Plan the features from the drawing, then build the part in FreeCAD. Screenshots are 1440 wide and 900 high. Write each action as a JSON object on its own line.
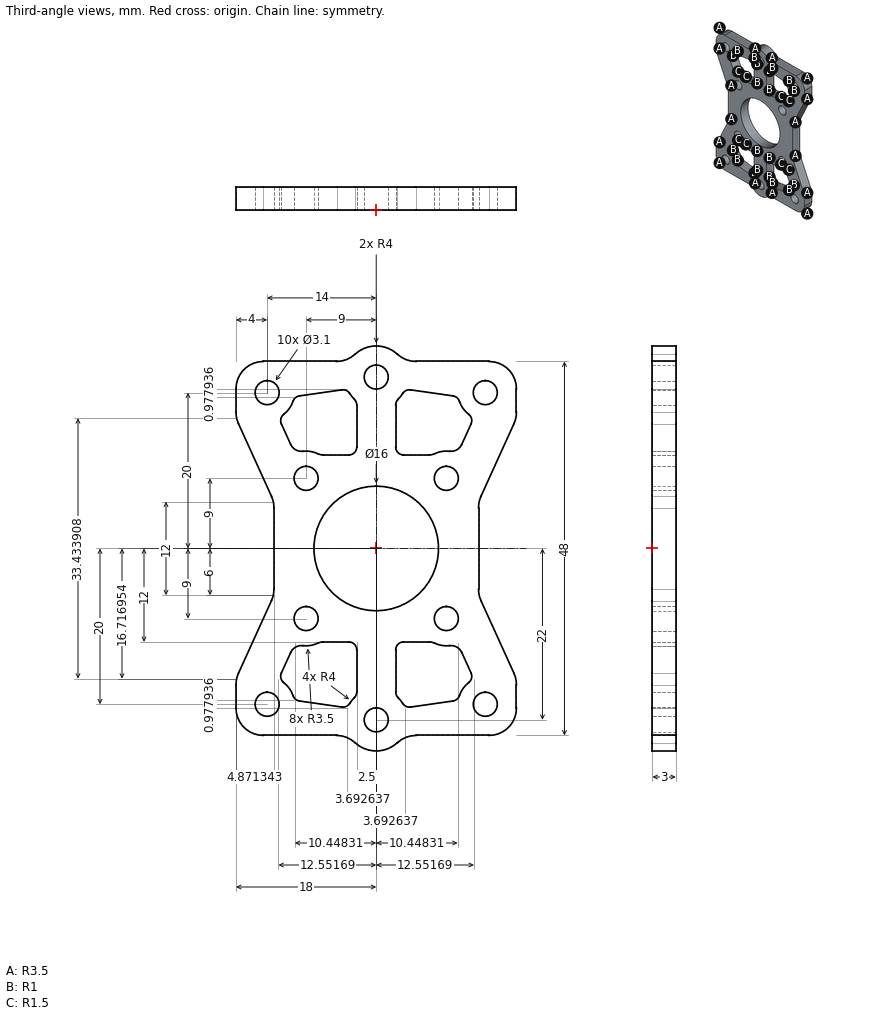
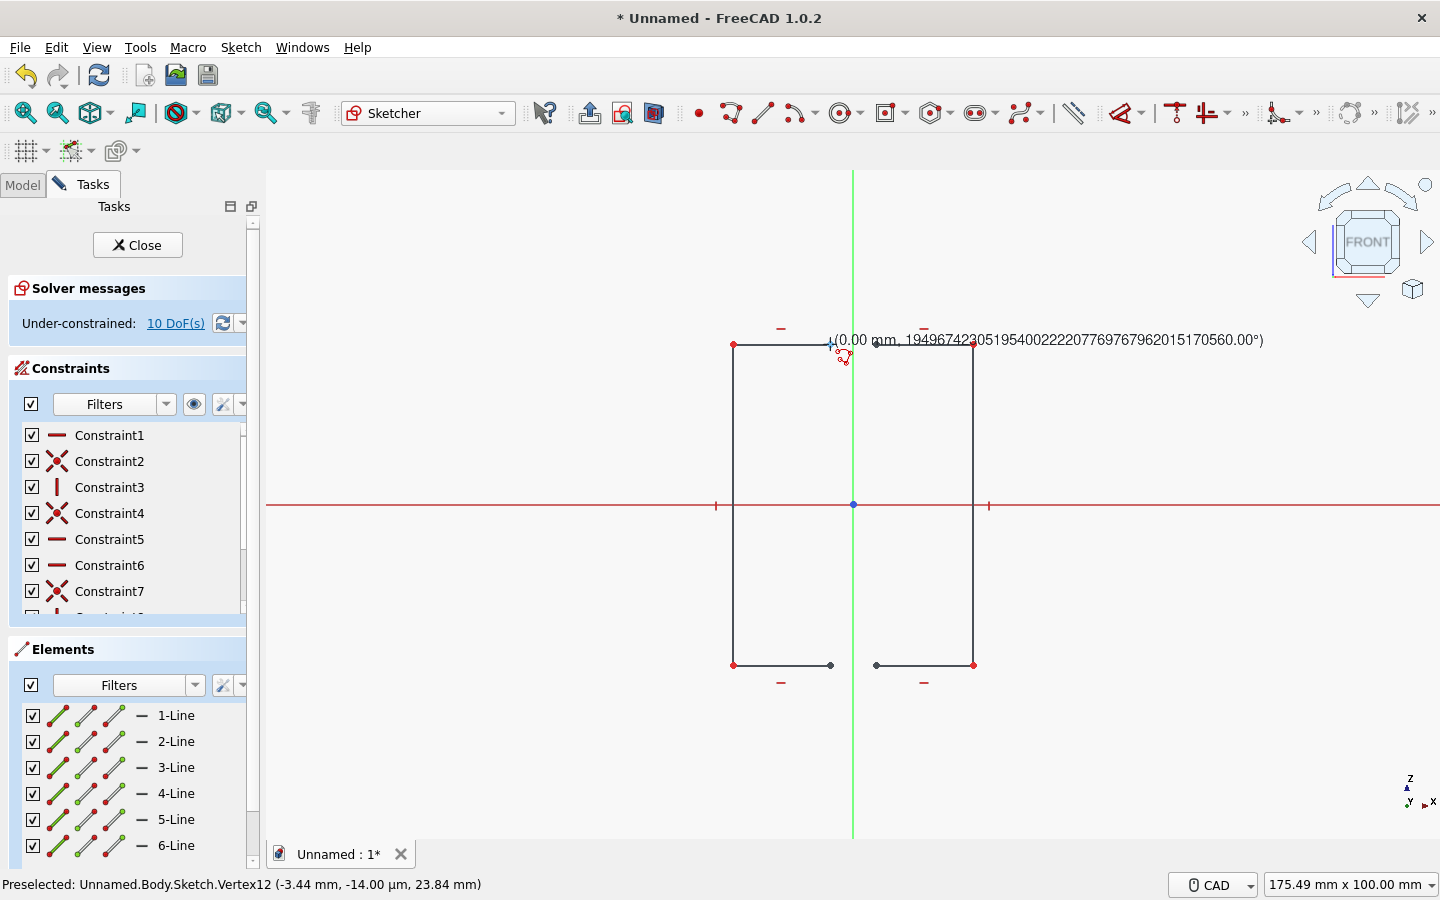
{"action": "key", "text": "g 3 a"}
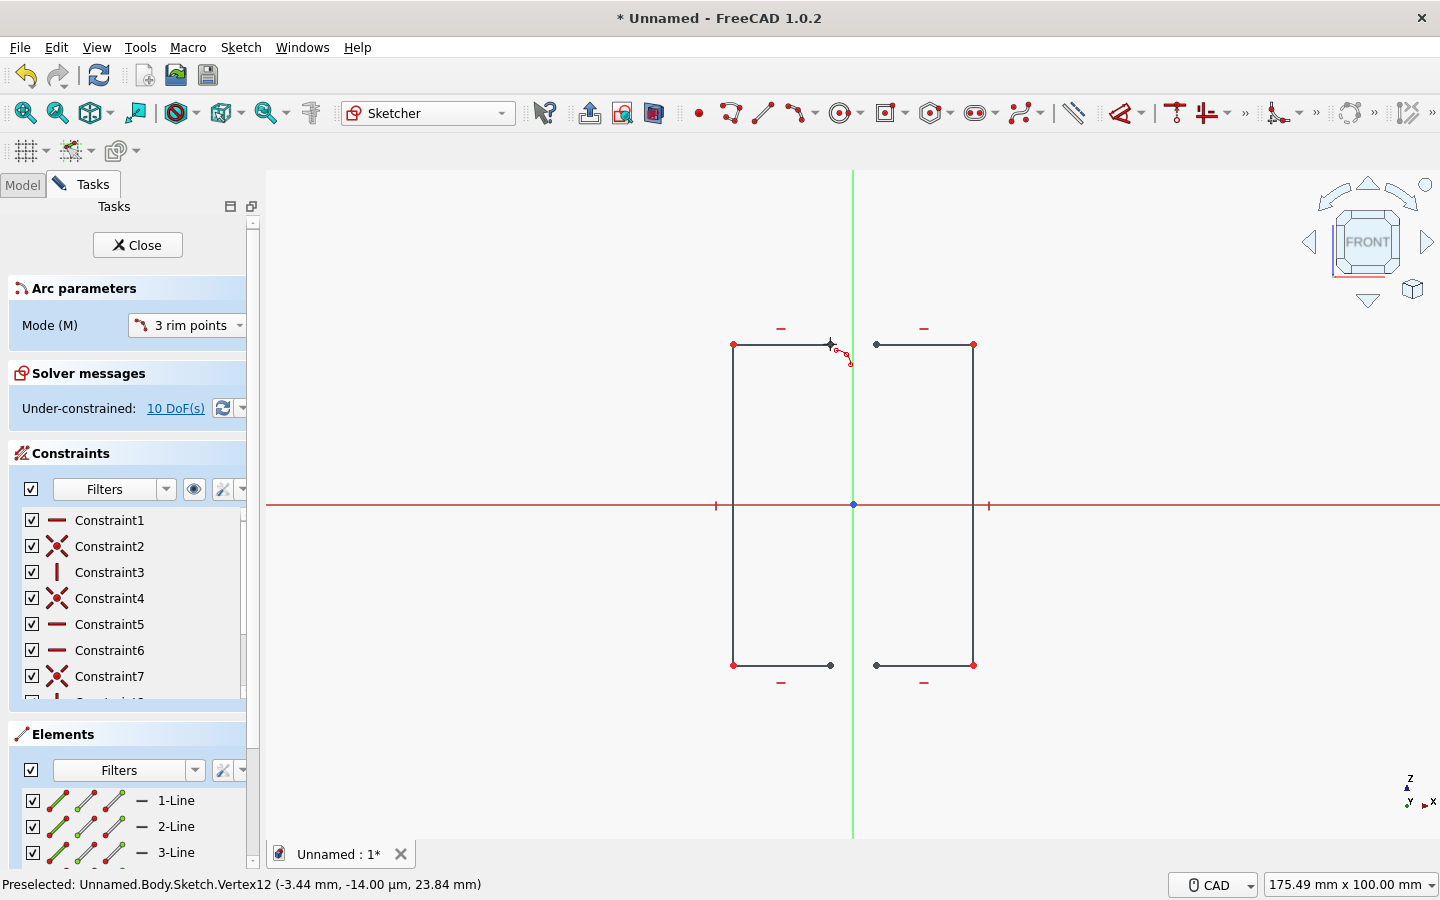
{"action": "left_click", "coordinate": [876, 666]}
{"action": "left_click", "coordinate": [830, 666]}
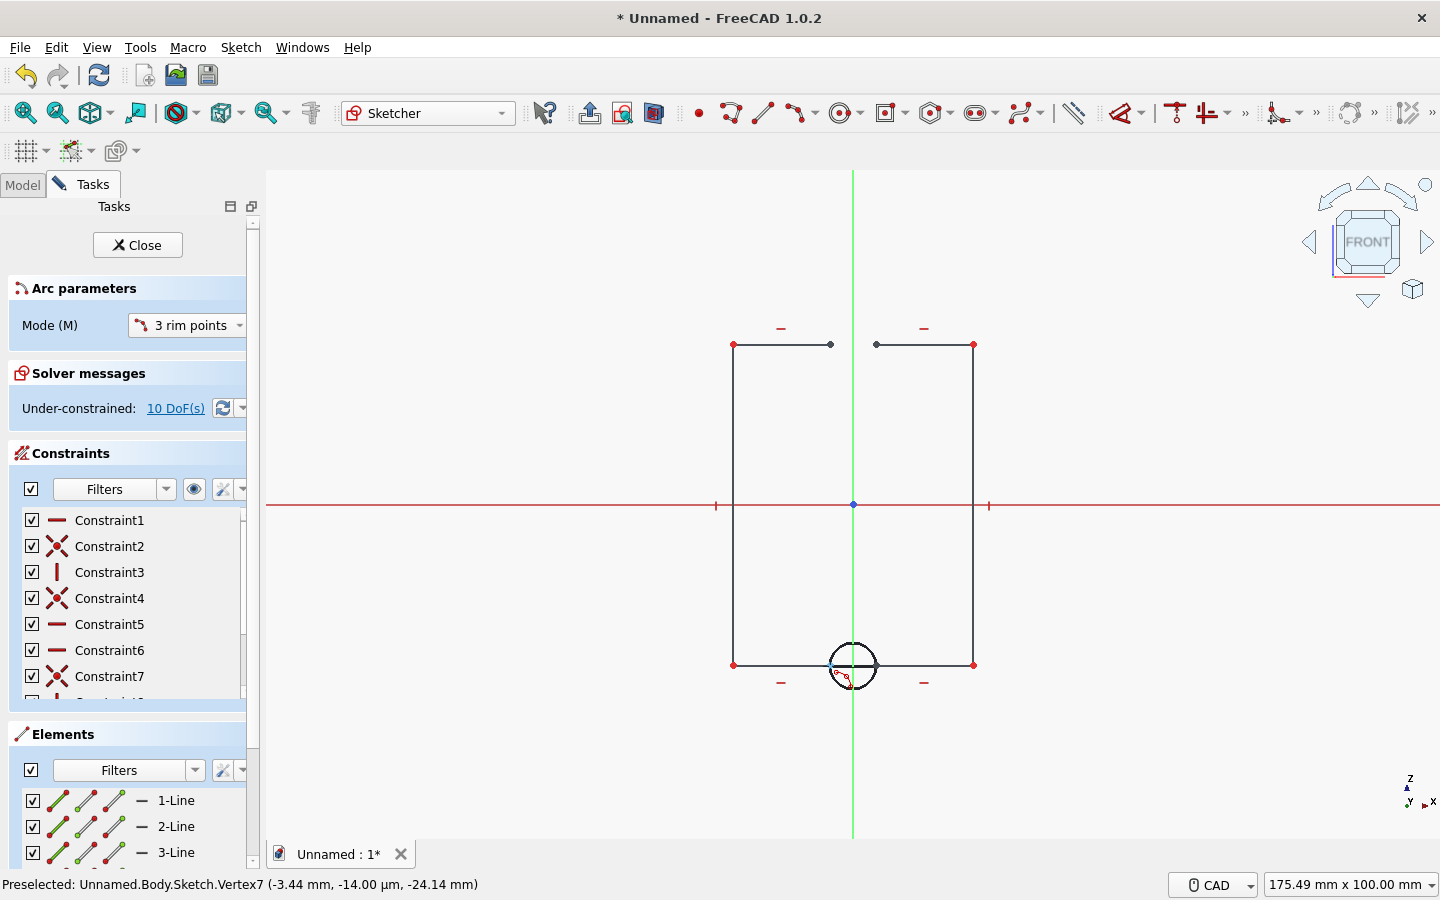
{"action": "scroll", "coordinate": [842, 676], "scroll_direction": "up", "scroll_amount": 2}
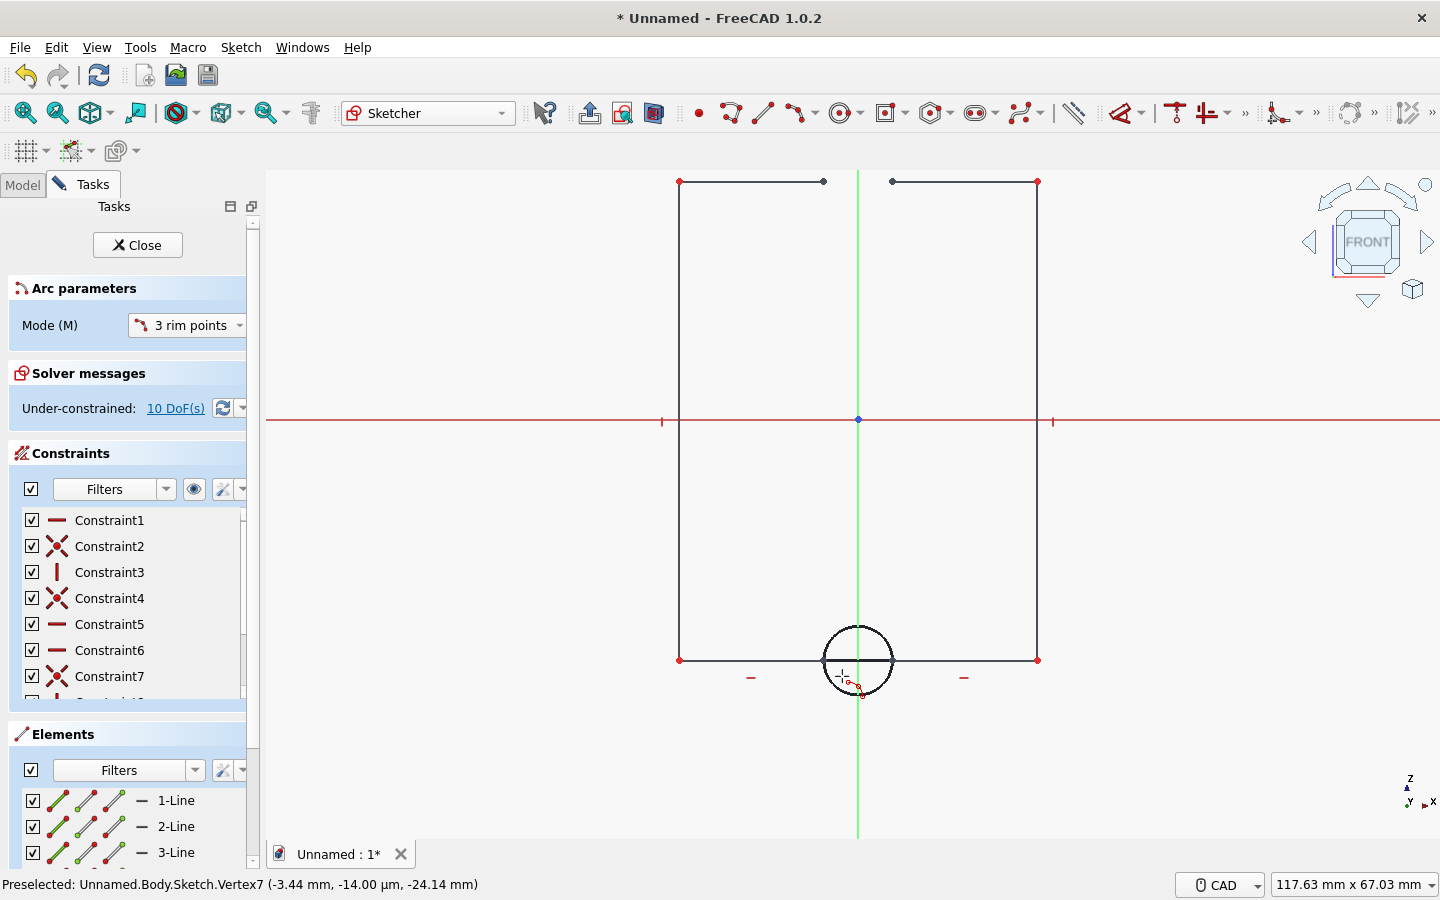
{"action": "left_click", "coordinate": [842, 676]}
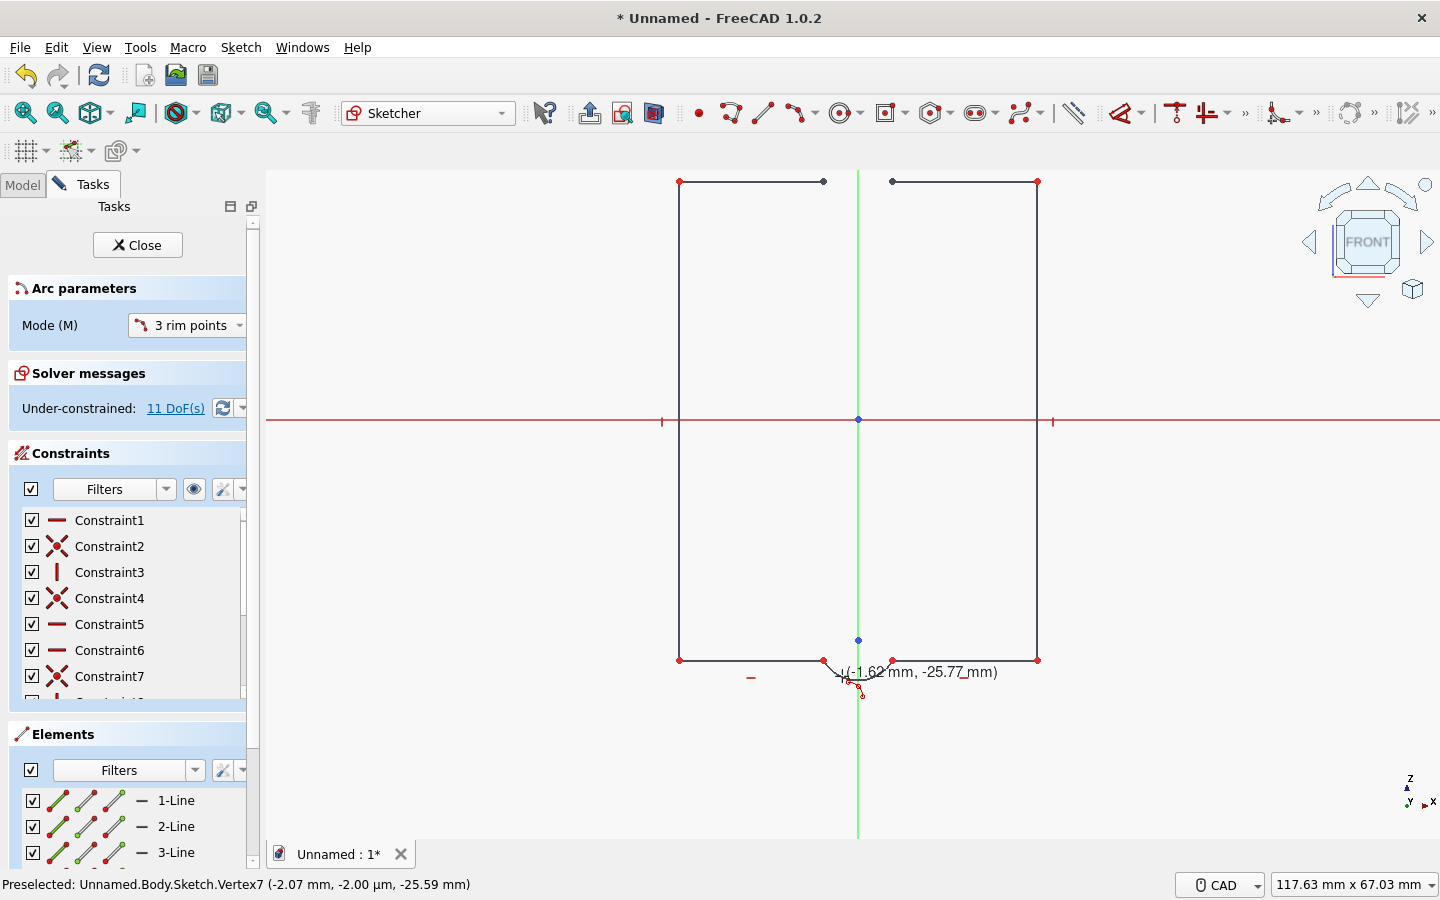
{"action": "scroll", "coordinate": [452, 811], "scroll_direction": "down", "scroll_amount": 1}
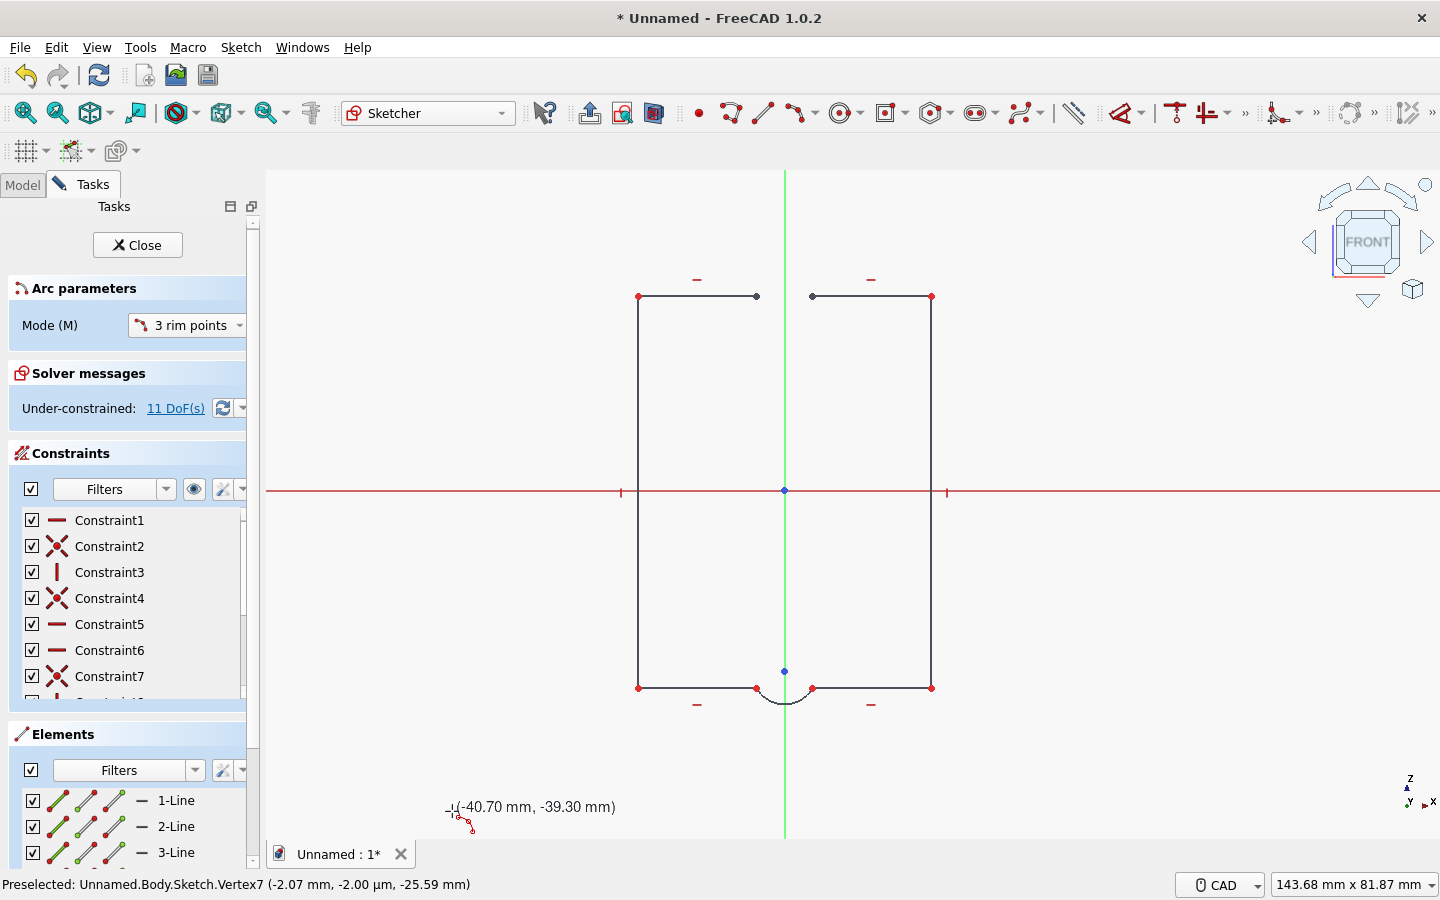
{"action": "left_click", "coordinate": [756, 296]}
{"action": "left_click", "coordinate": [813, 296]}
{"action": "left_click", "coordinate": [798, 281]}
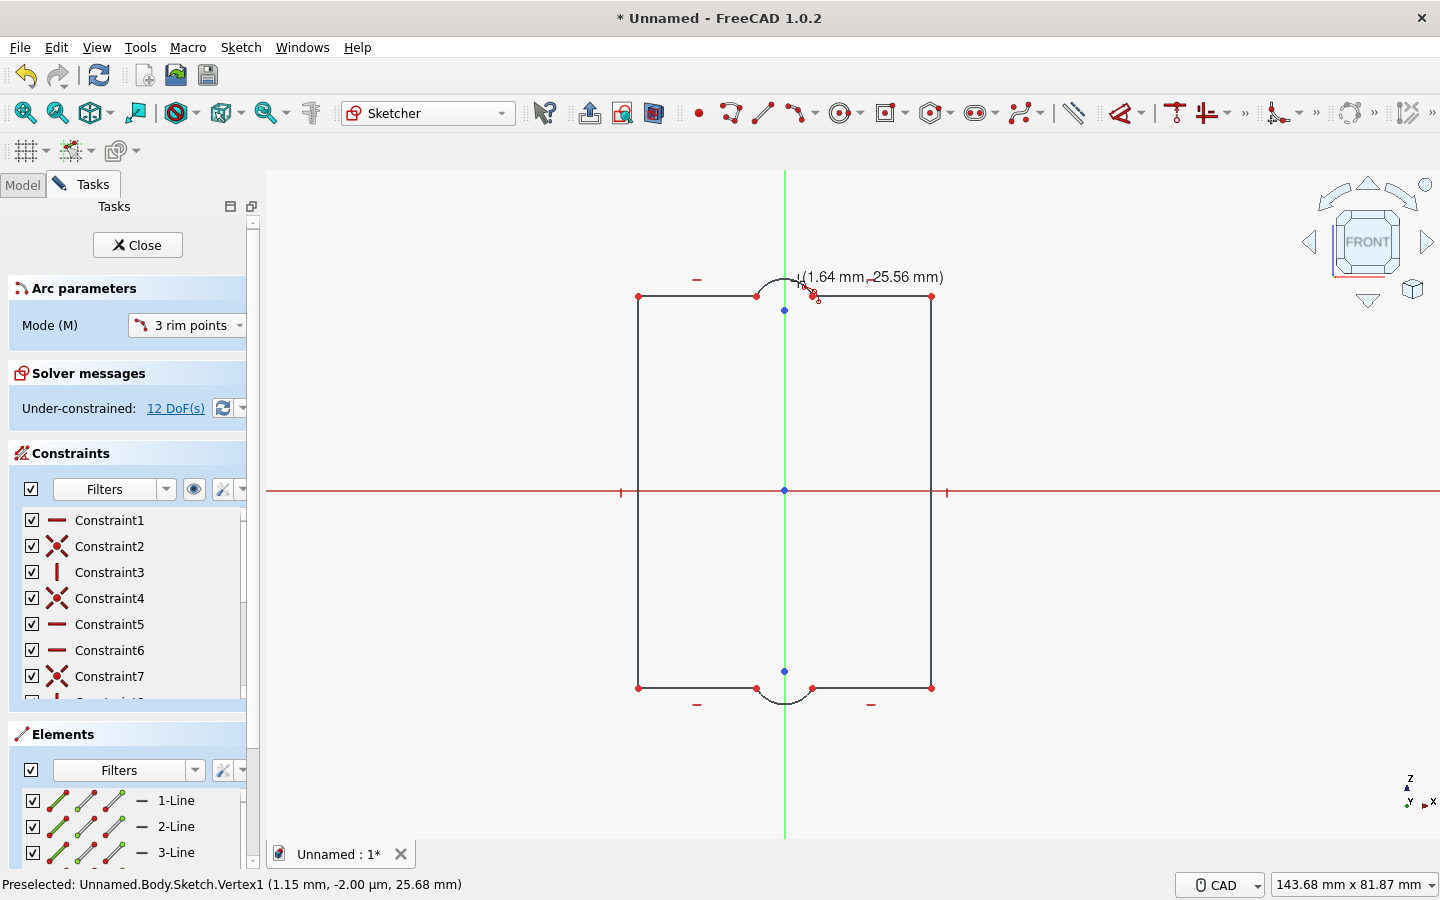
{"action": "left_click", "coordinate": [840, 114]}